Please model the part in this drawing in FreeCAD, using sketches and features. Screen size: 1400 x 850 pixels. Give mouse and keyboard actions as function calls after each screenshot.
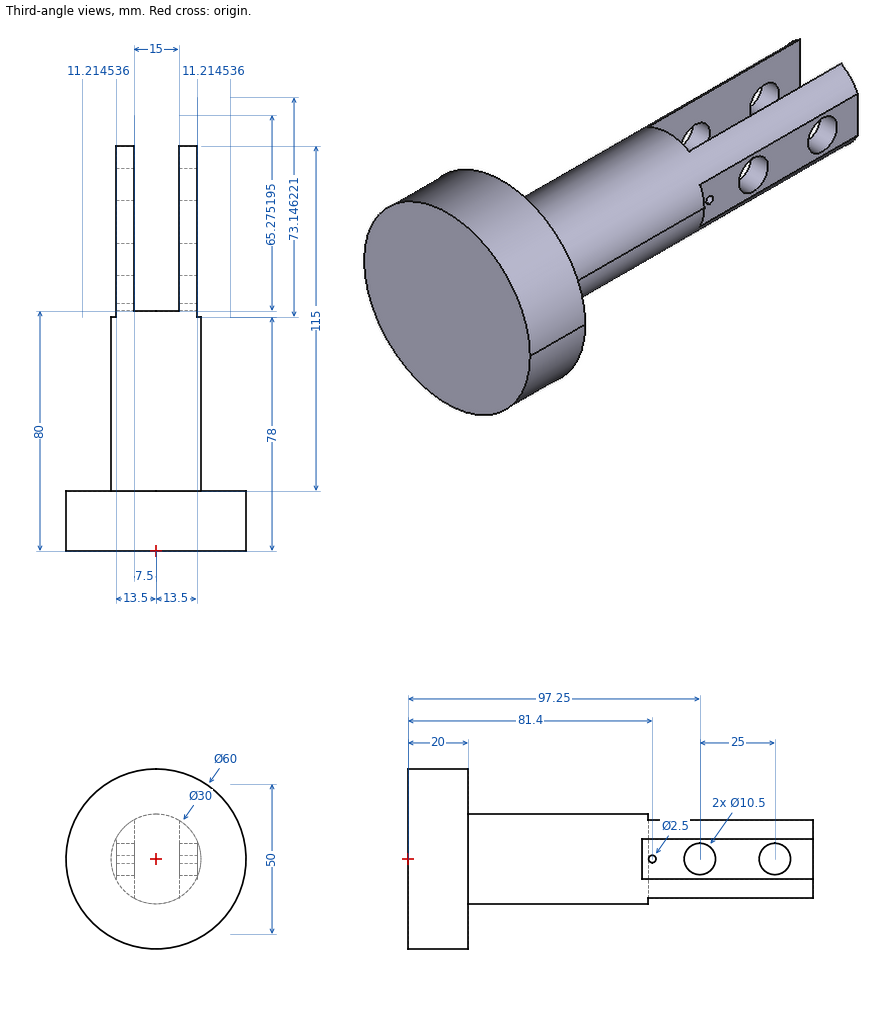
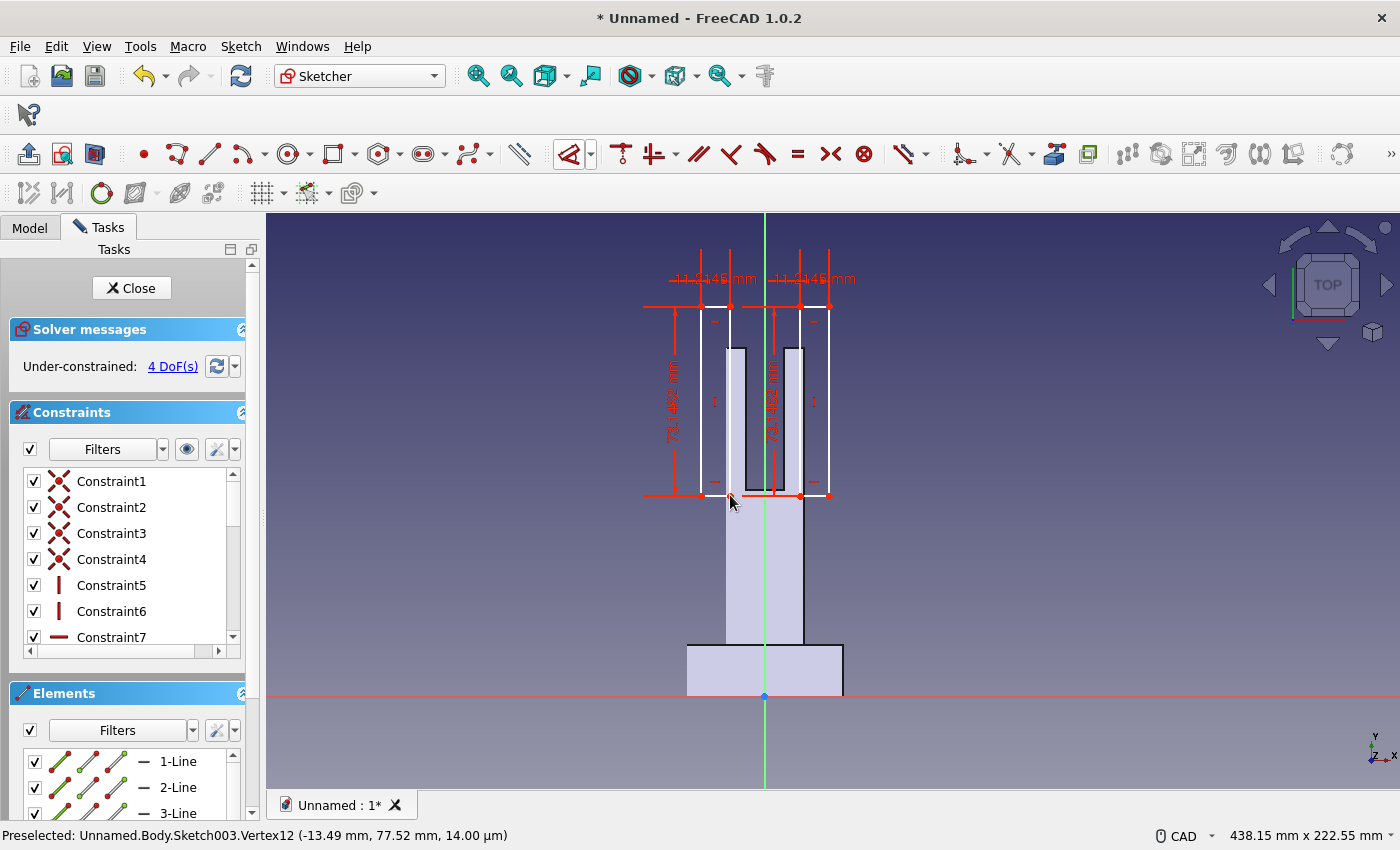
click(800, 496)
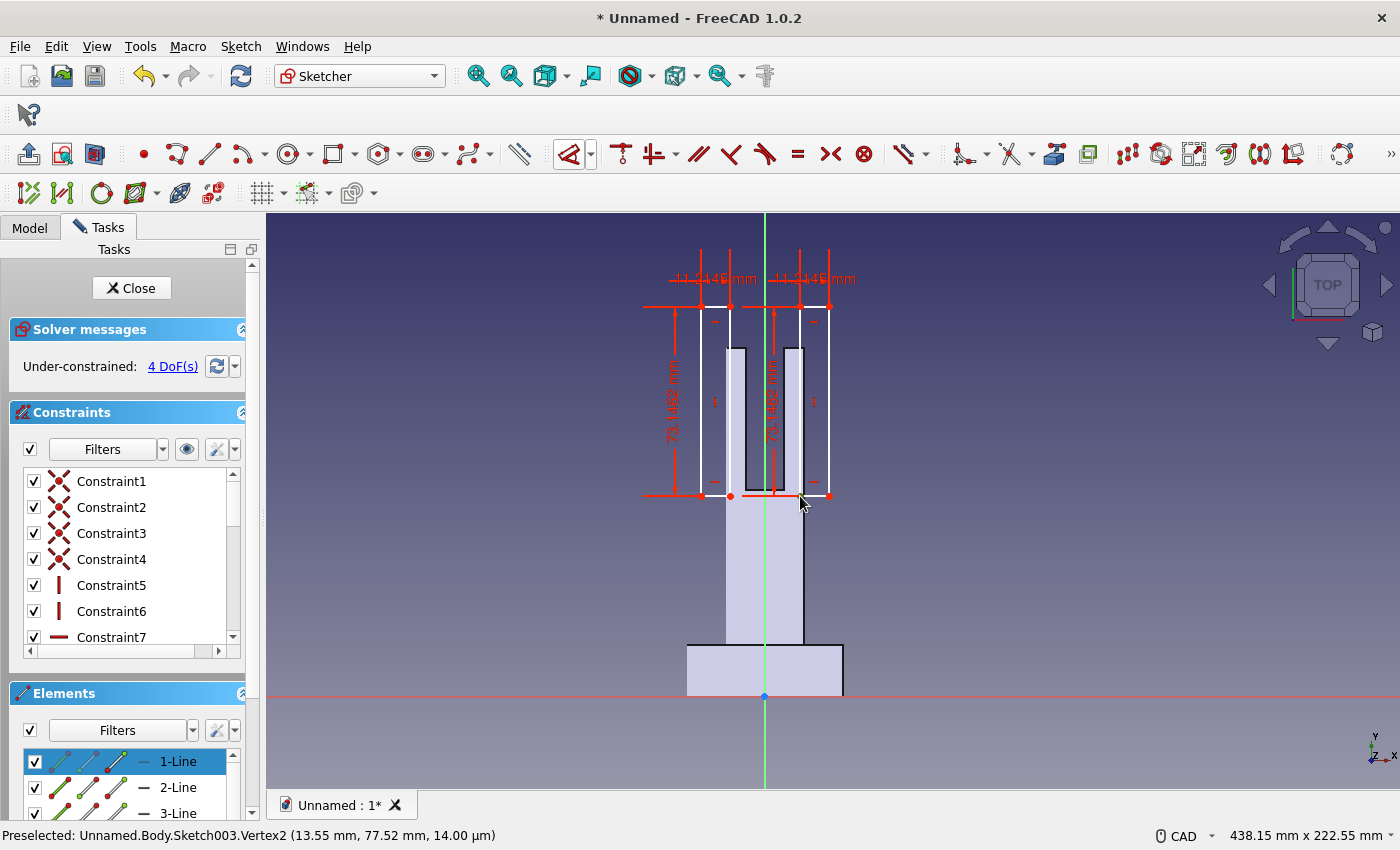
key(i)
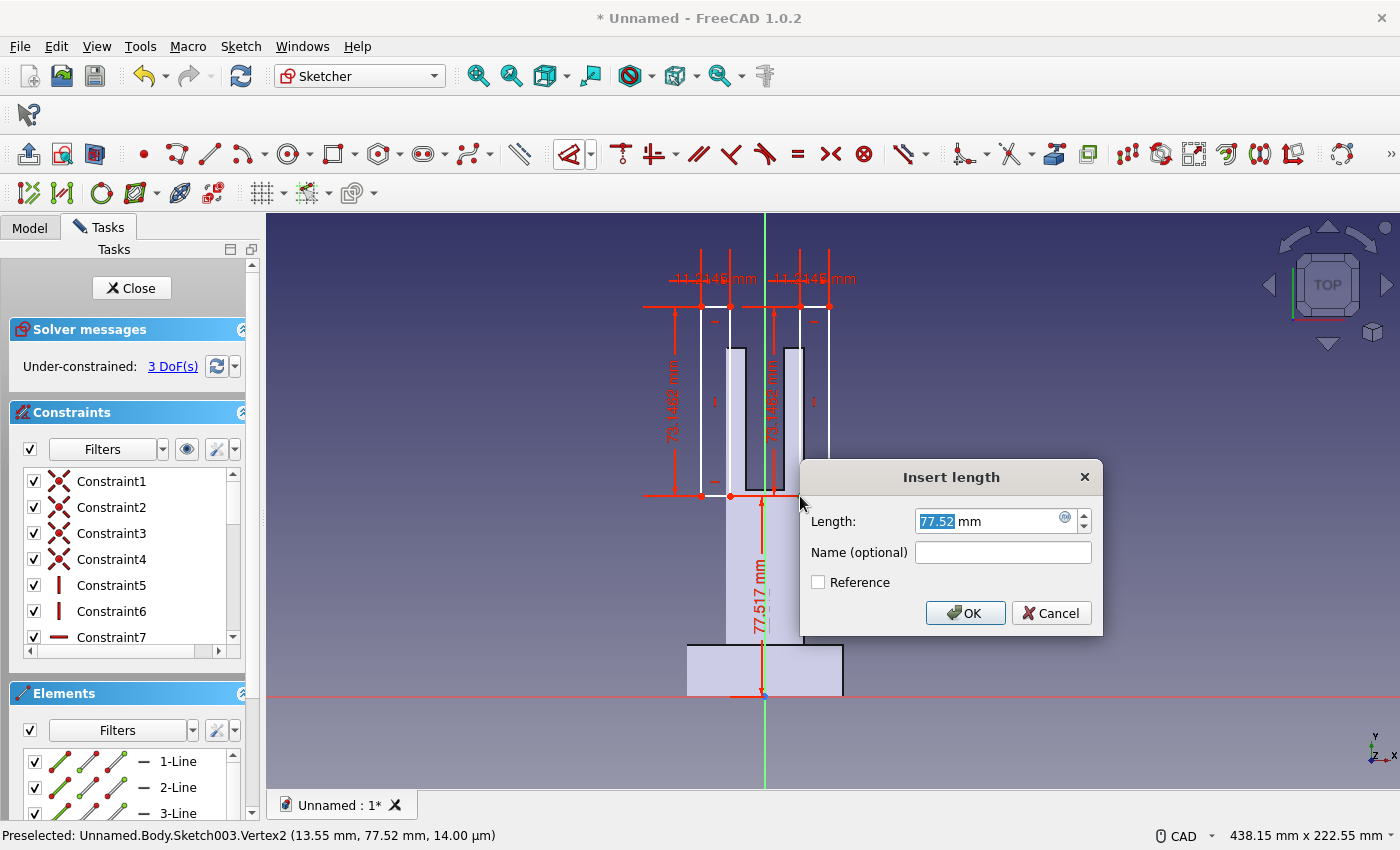
text(78)
key(Return)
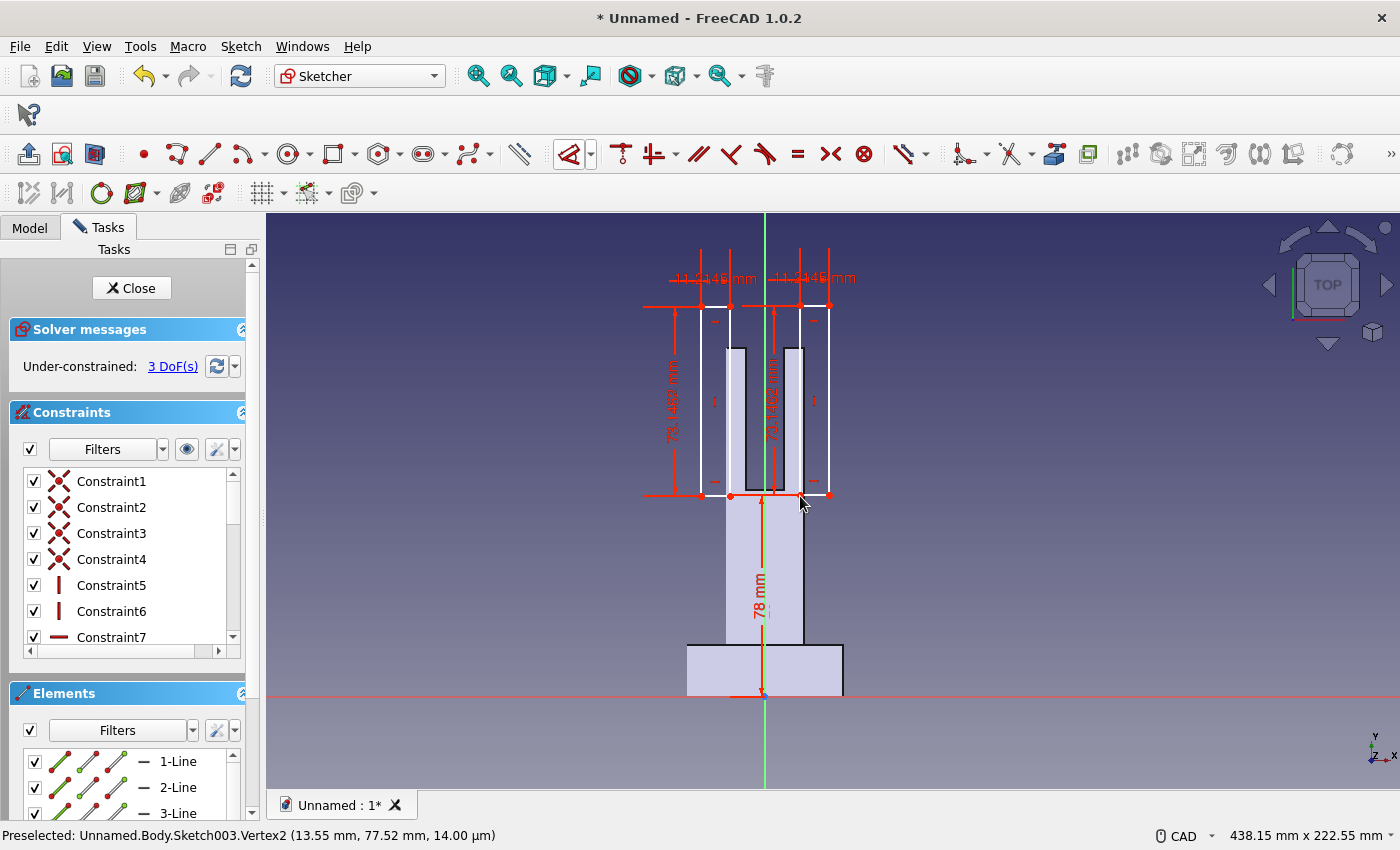
click(701, 496)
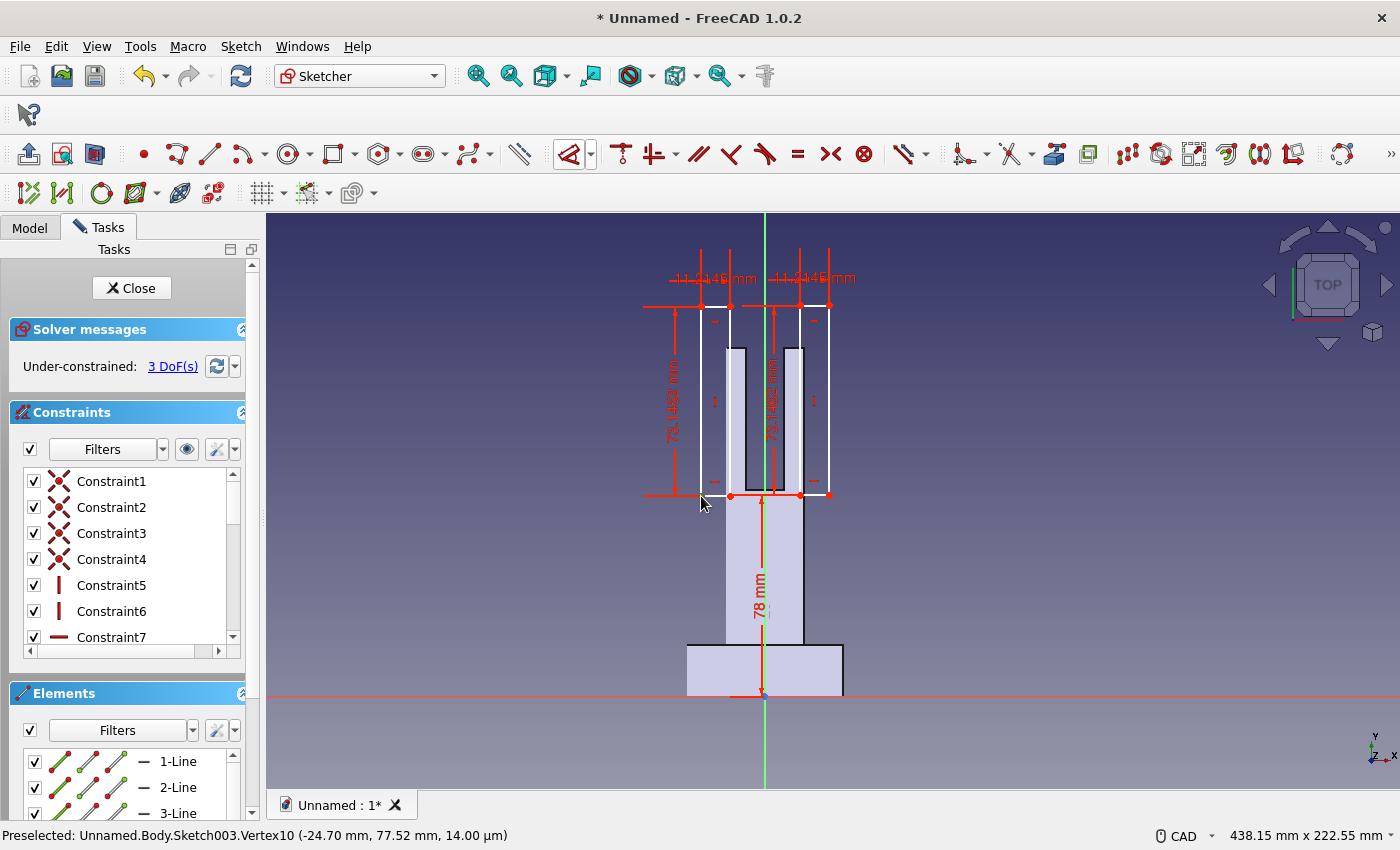
key(i)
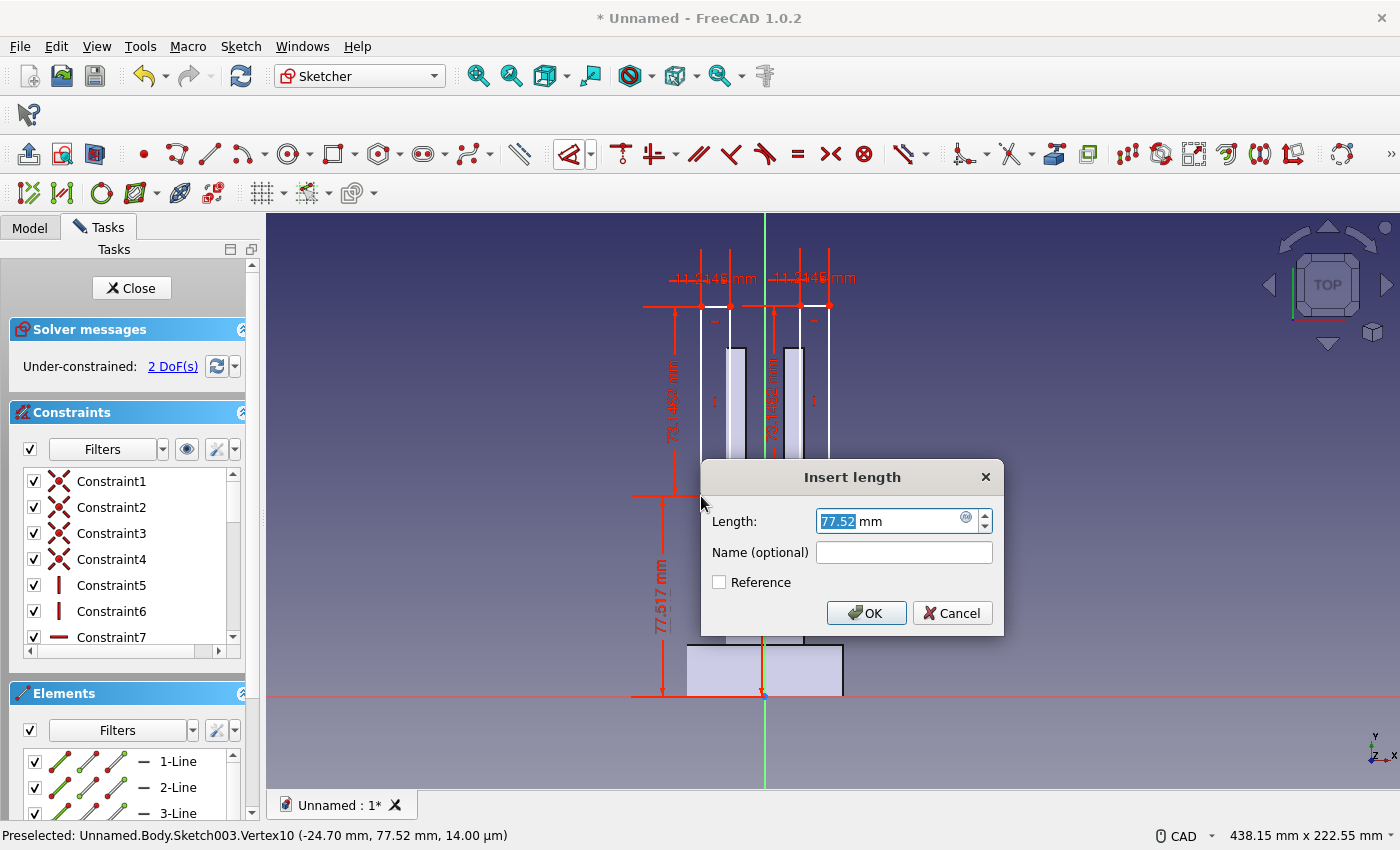
text(78)
key(Return)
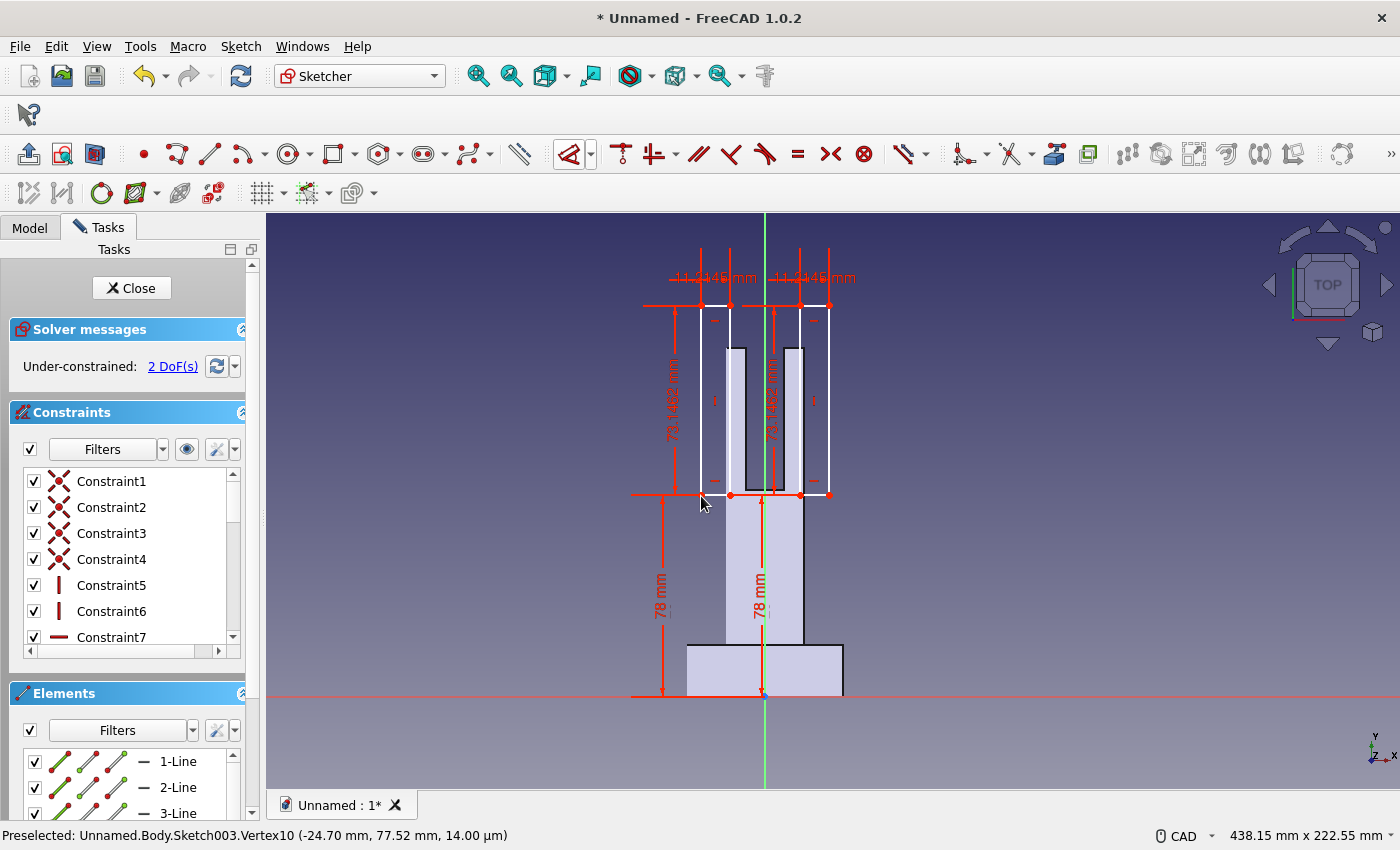
click(800, 306)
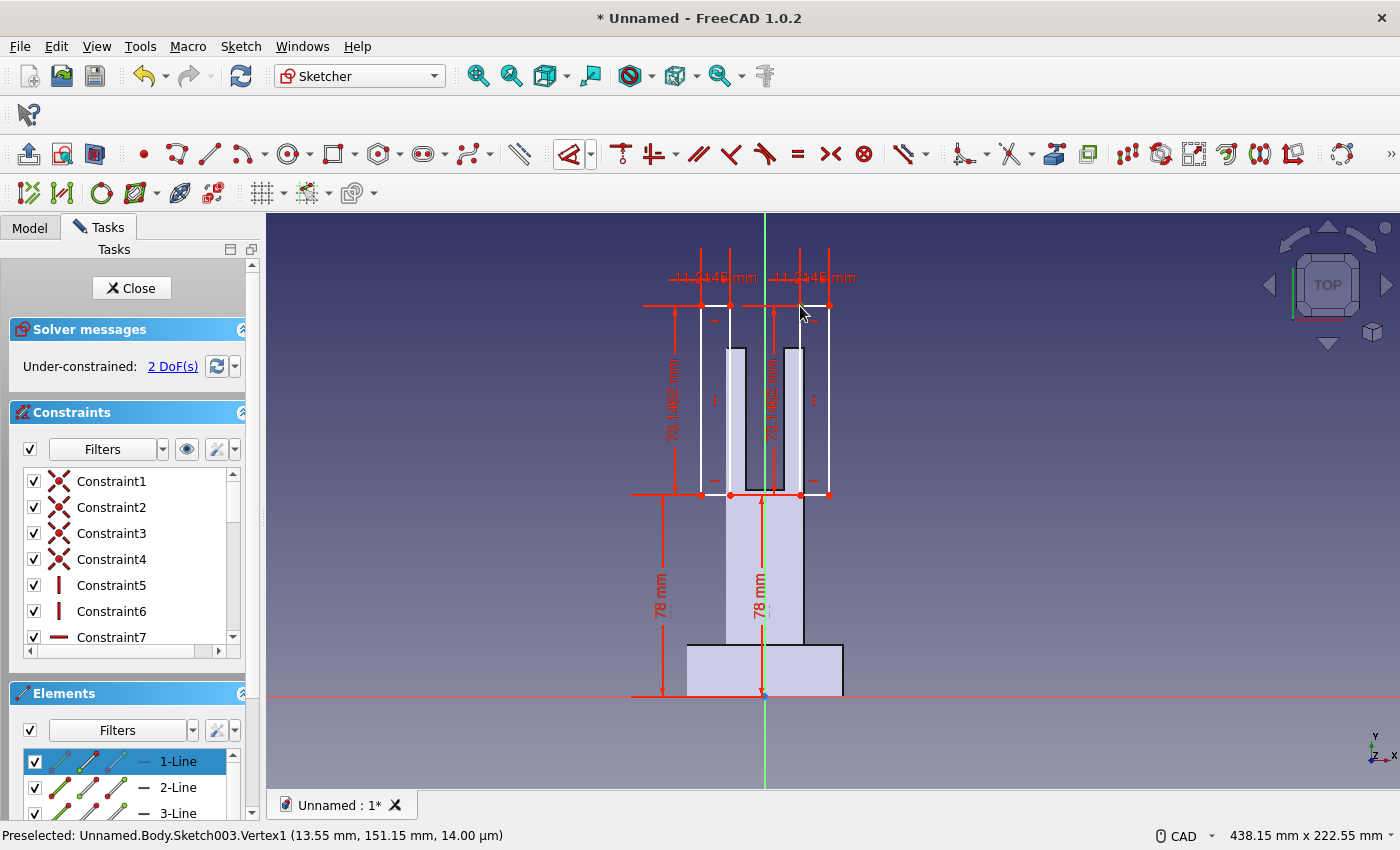
key(l)